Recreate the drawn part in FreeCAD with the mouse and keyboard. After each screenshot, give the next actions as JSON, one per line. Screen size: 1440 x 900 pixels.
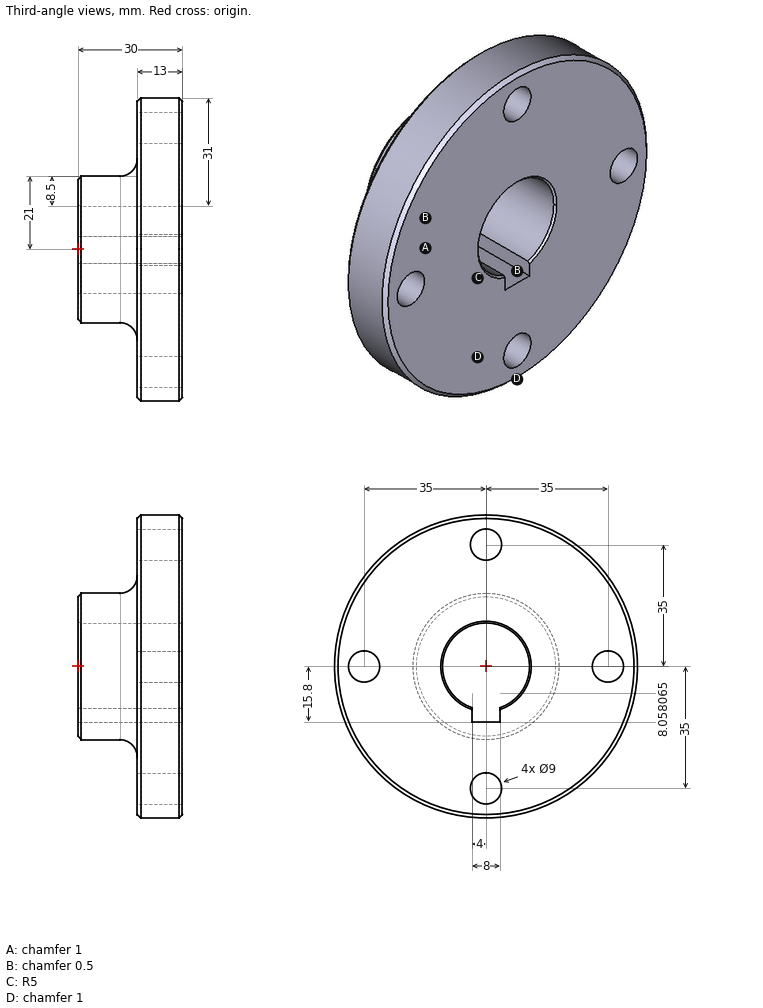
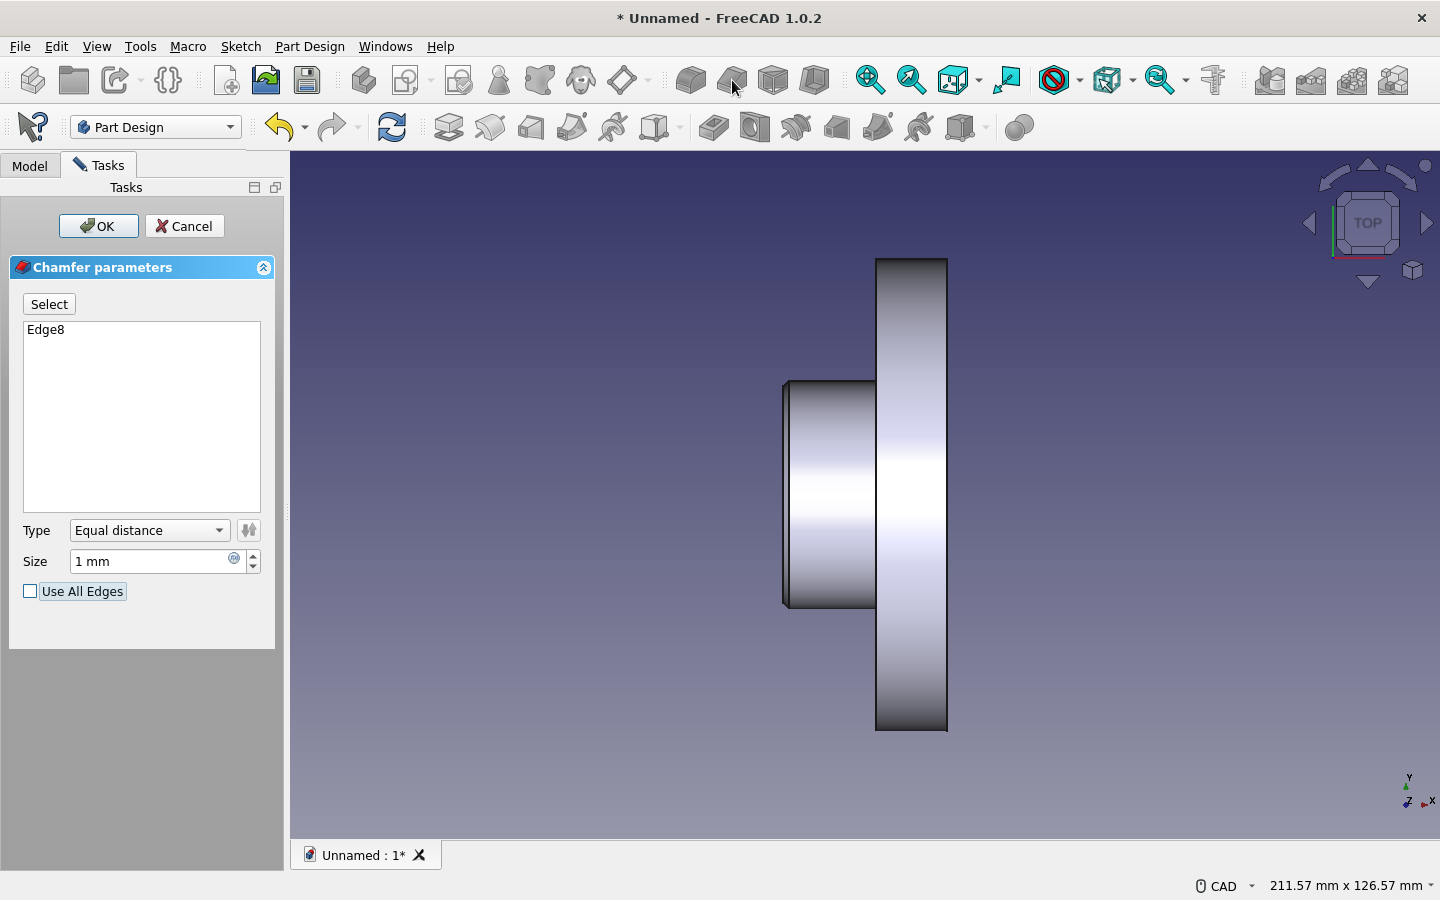
{"action": "left_click", "coordinate": [99, 226]}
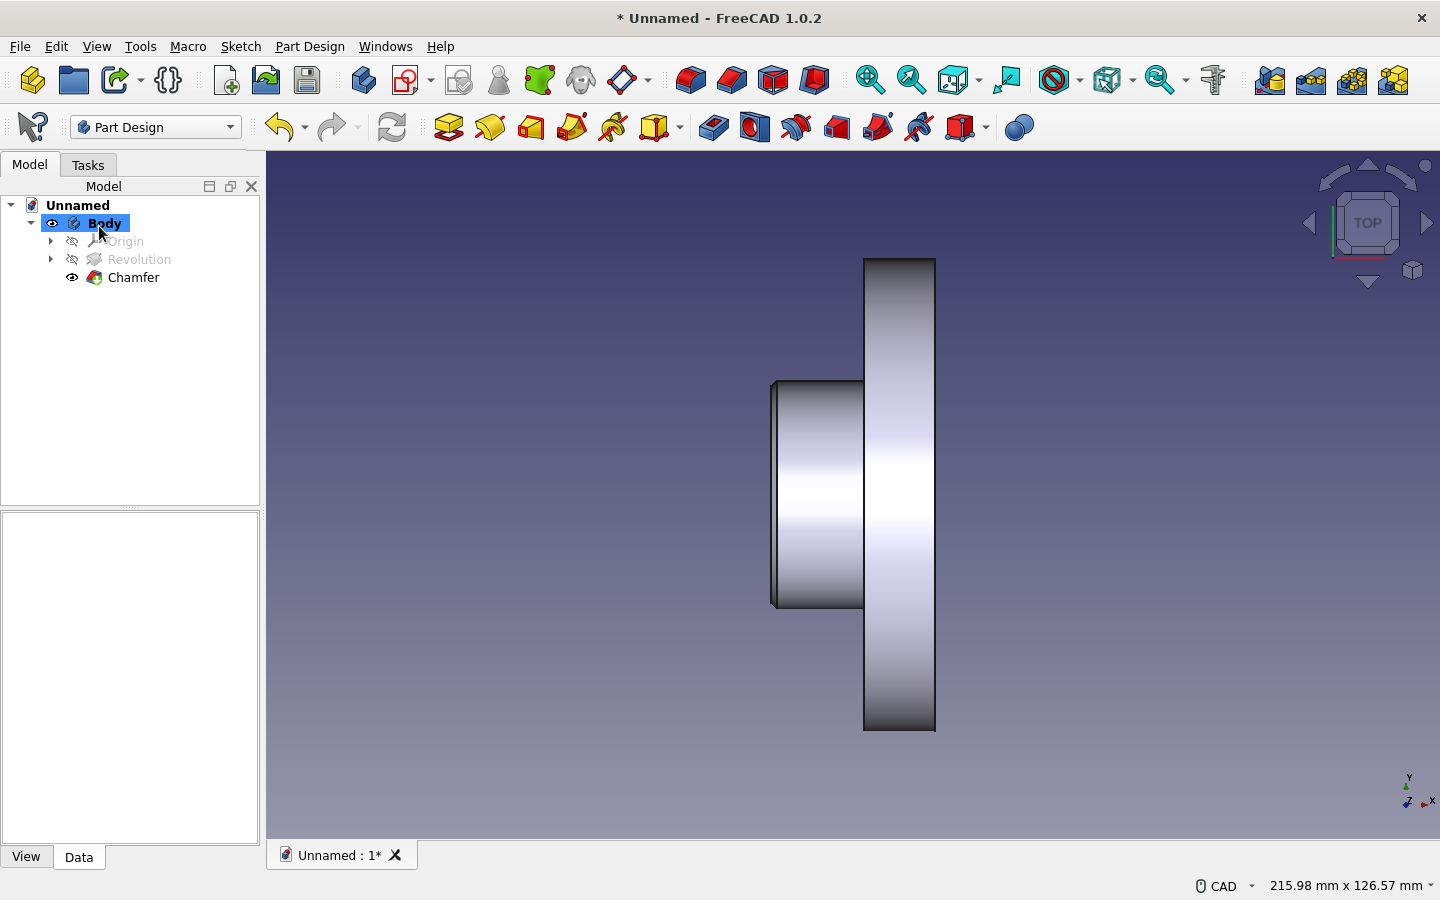
{"action": "key", "text": "0"}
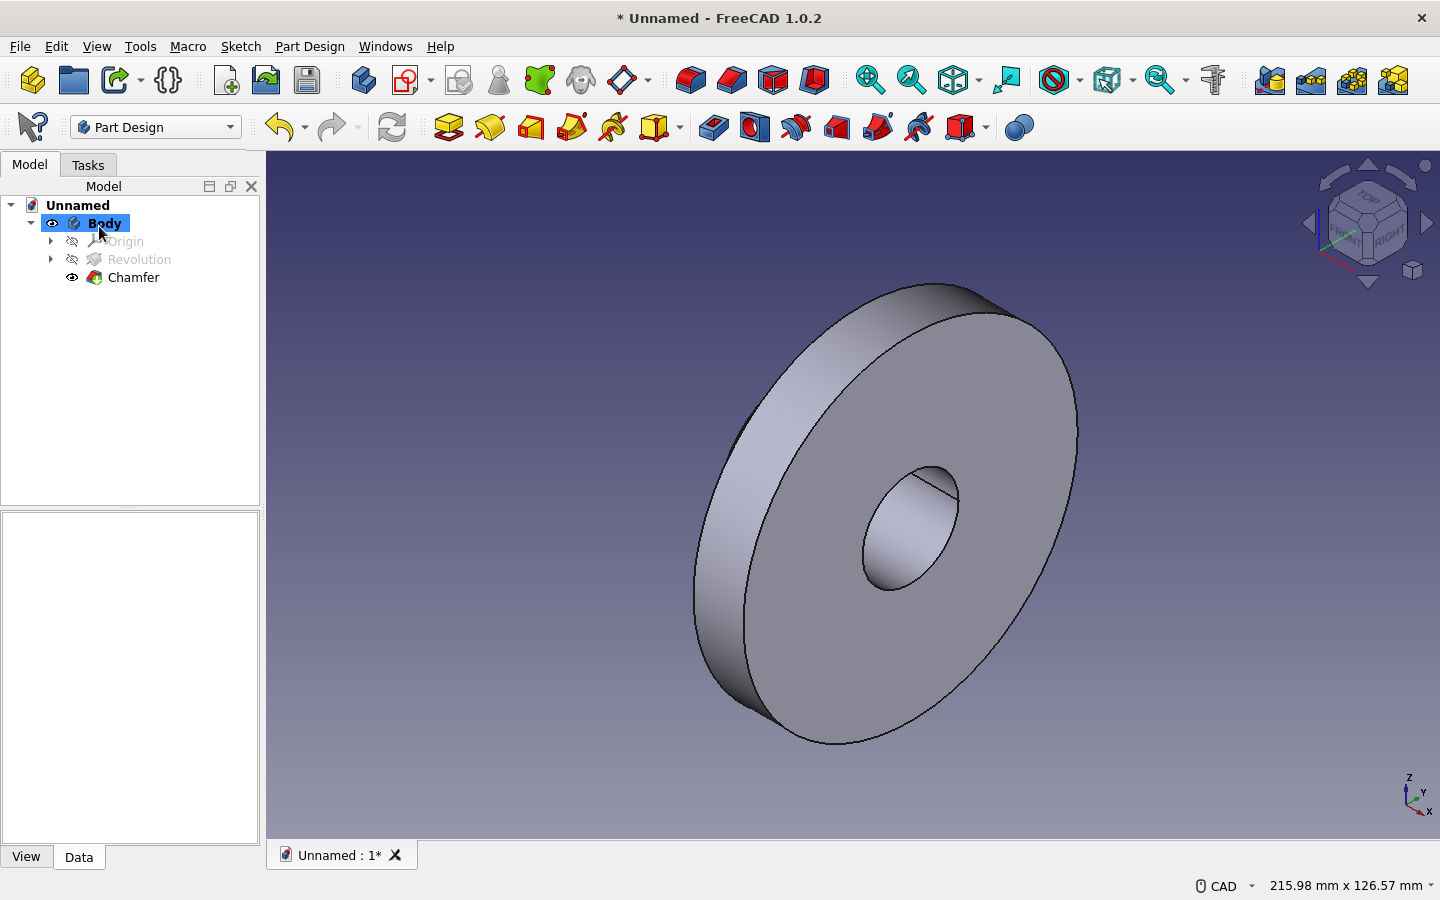
{"action": "left_click", "coordinate": [896, 589]}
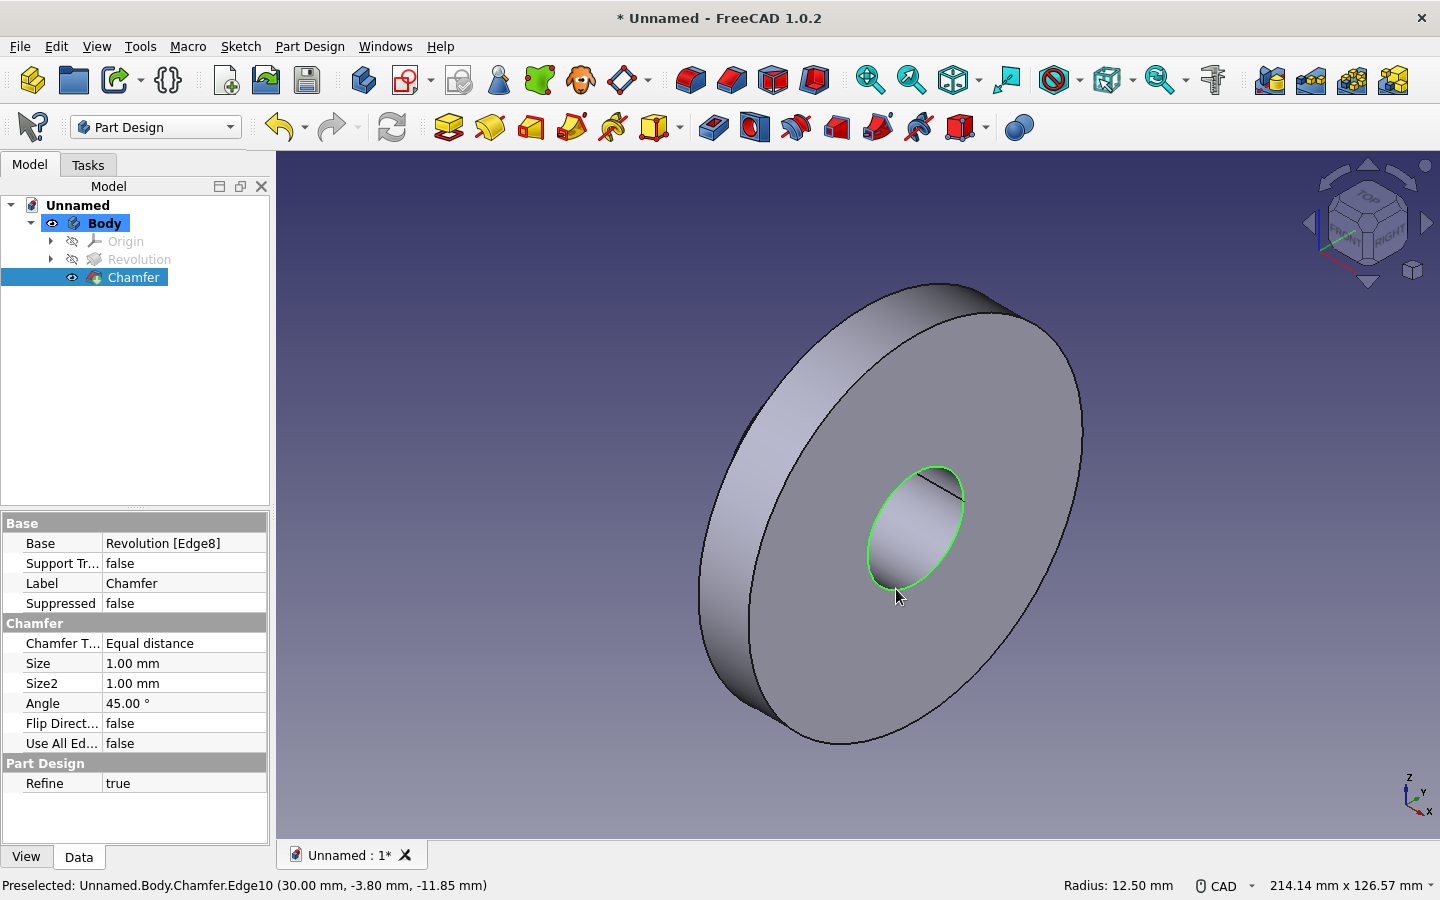
{"action": "key", "text": "2"}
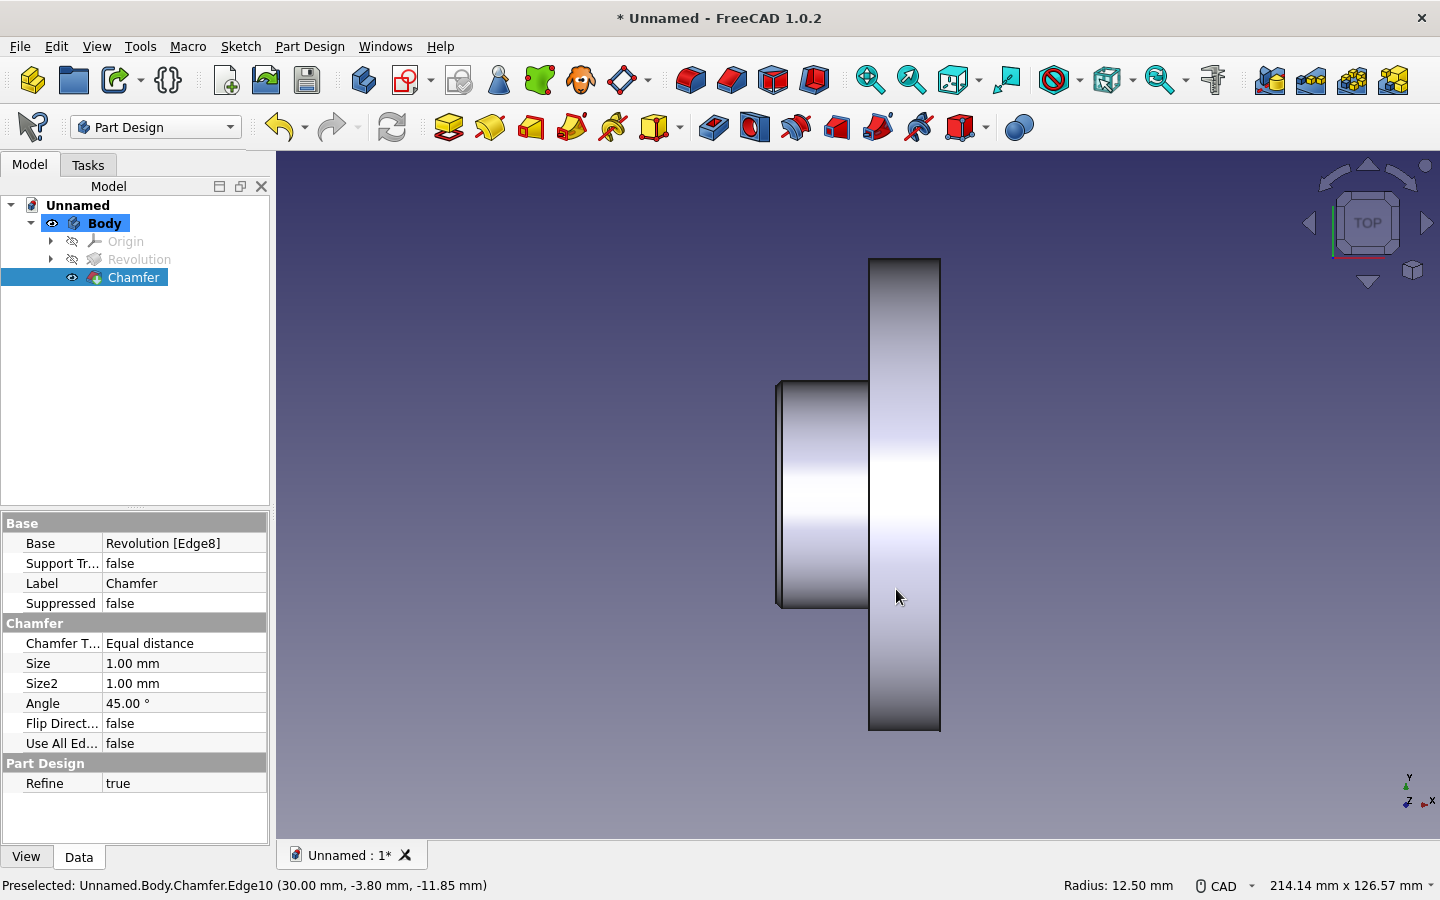
{"action": "key", "text": "1"}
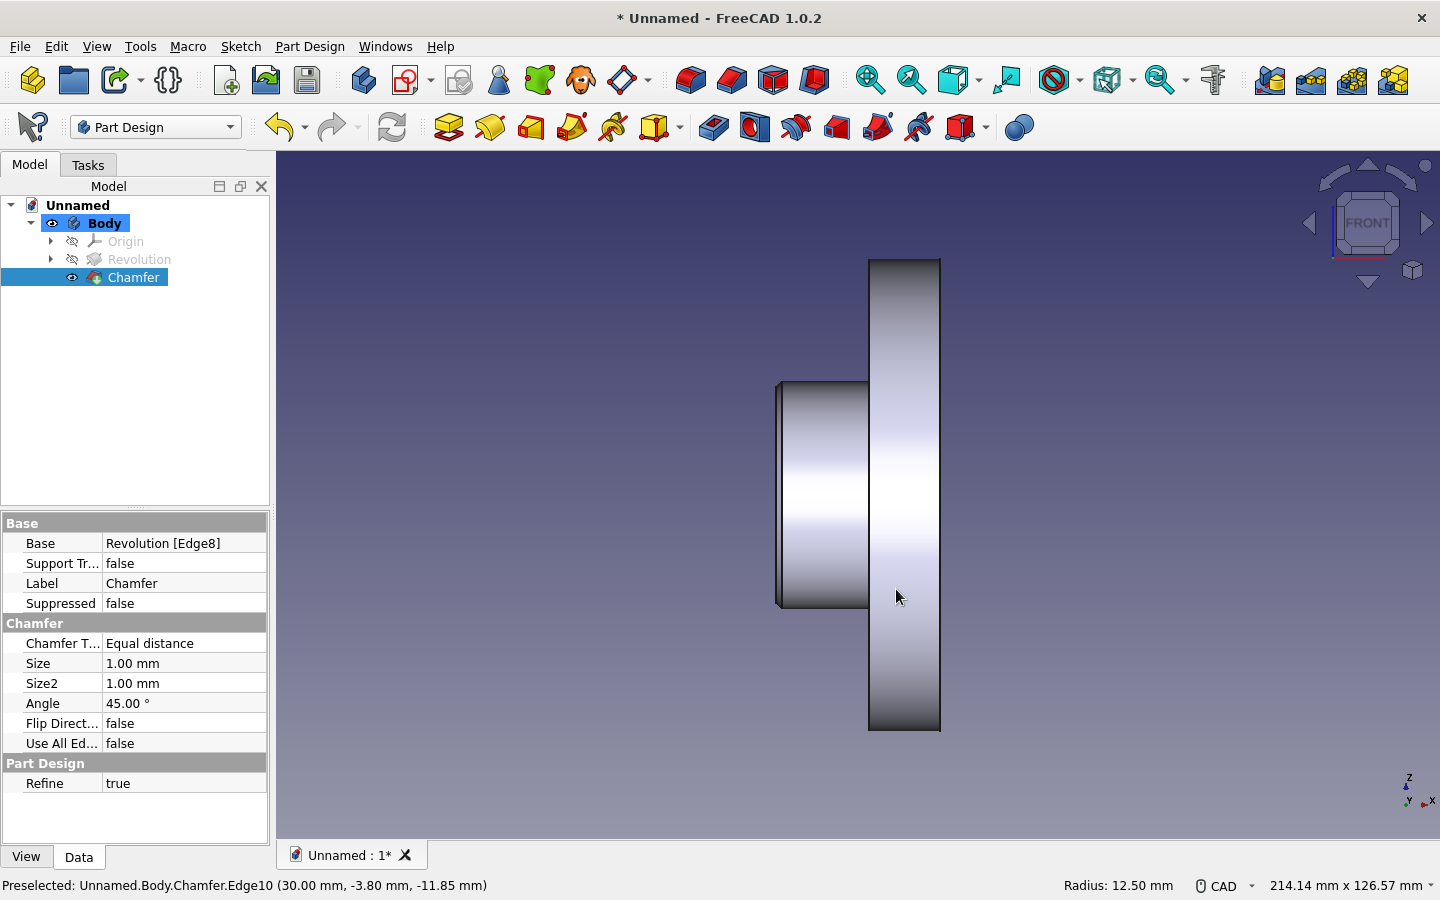
{"action": "key", "text": "3"}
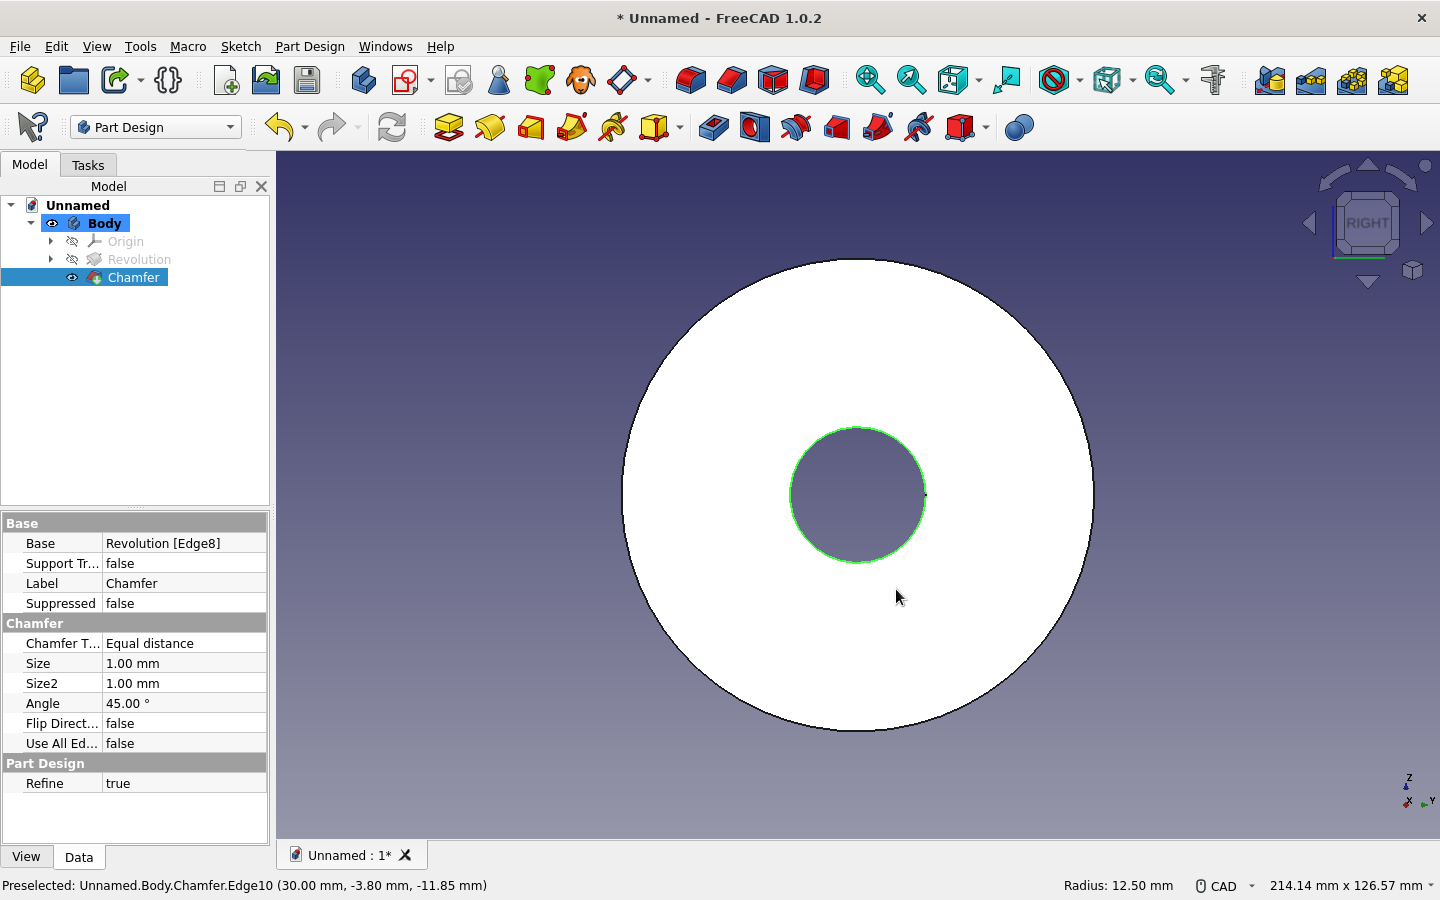
{"action": "key", "text": "5"}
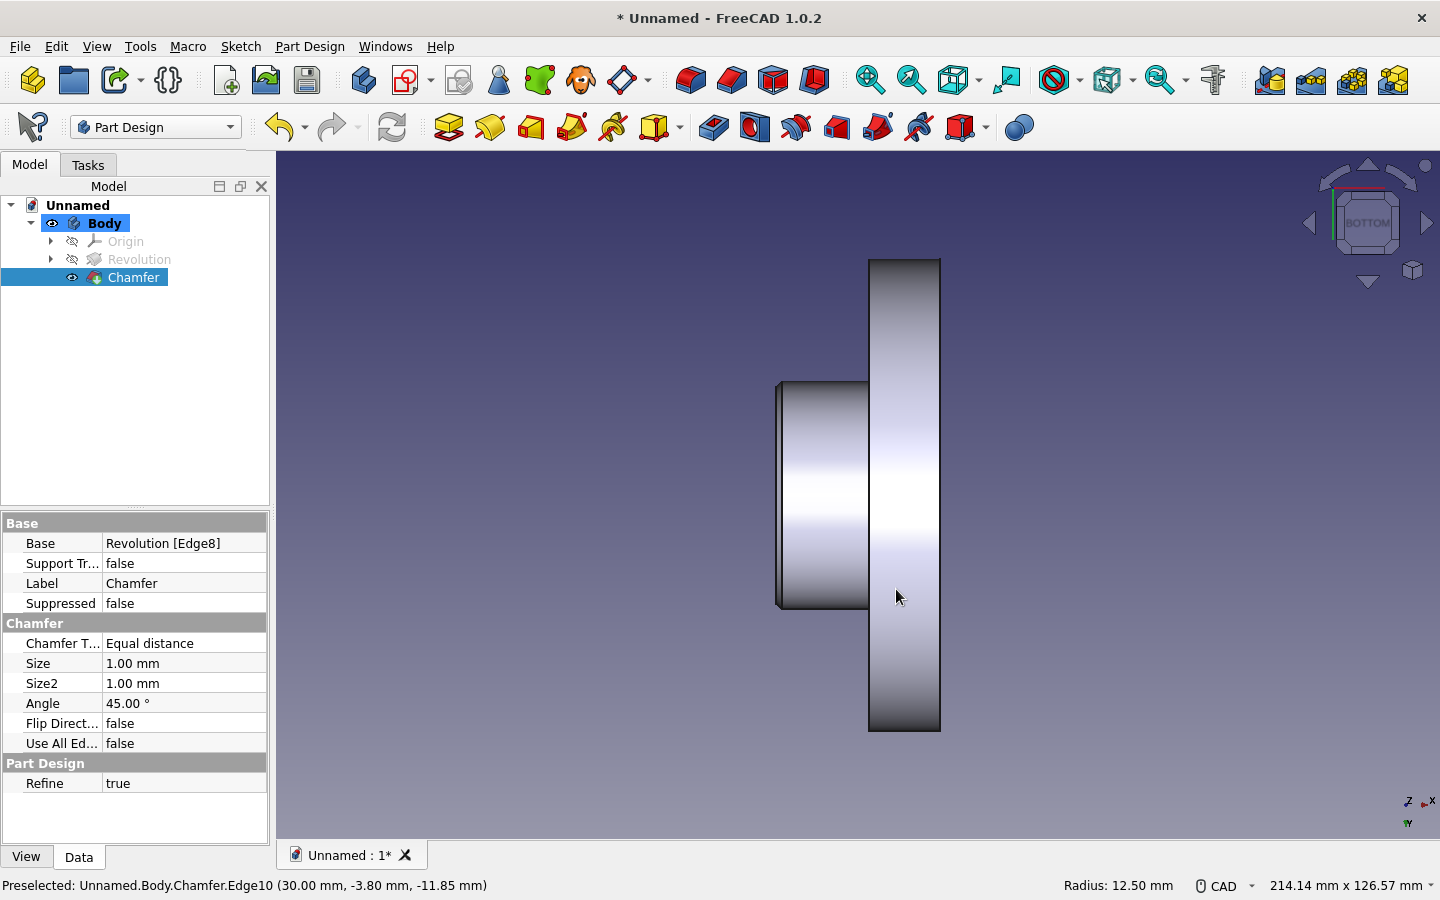
{"action": "key", "text": "4"}